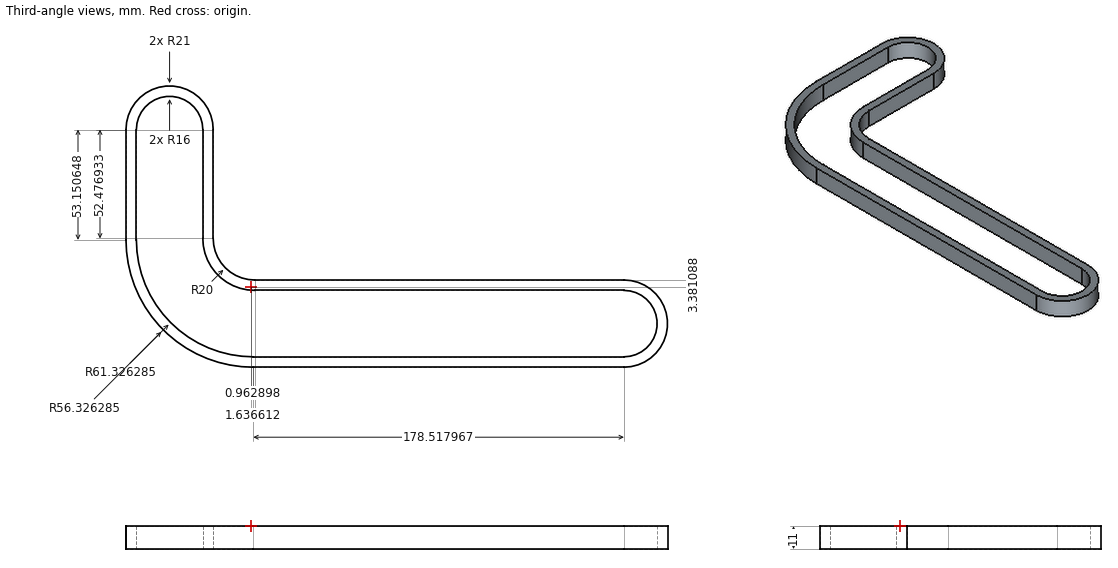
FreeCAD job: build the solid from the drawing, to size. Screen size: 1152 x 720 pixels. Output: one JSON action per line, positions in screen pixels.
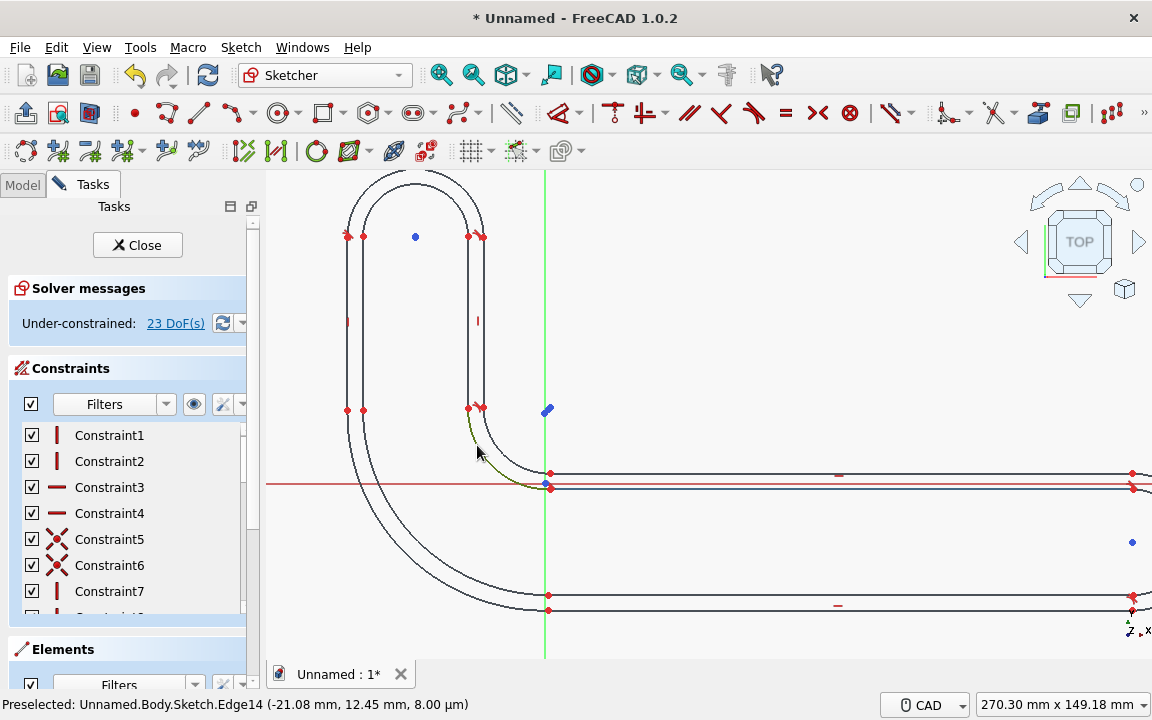
{"action": "left_click", "coordinate": [754, 114]}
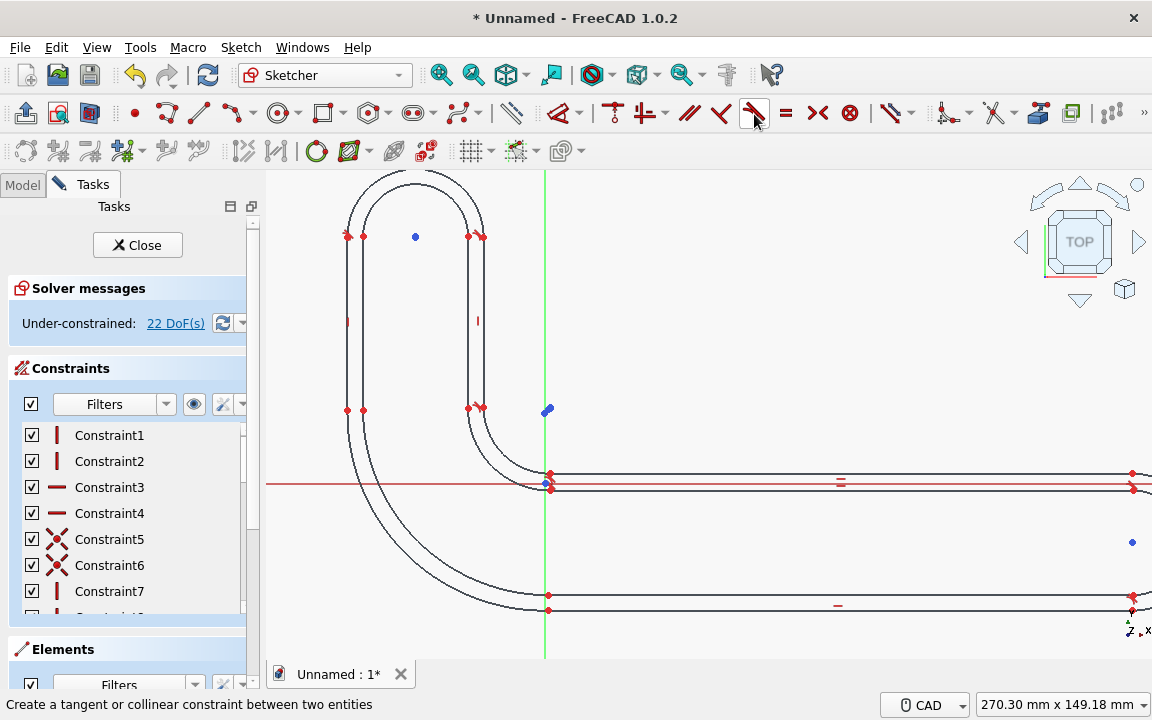
{"action": "scroll", "coordinate": [725, 491], "scroll_direction": "up", "scroll_amount": 4}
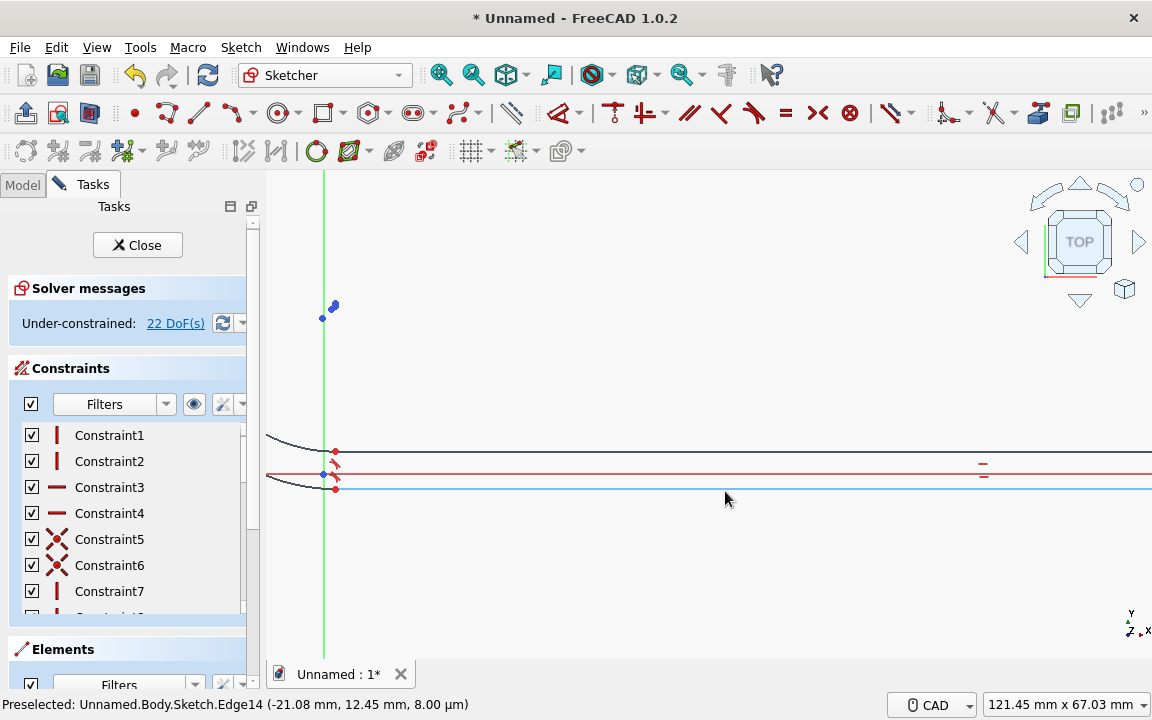
{"action": "left_click", "coordinate": [725, 489]}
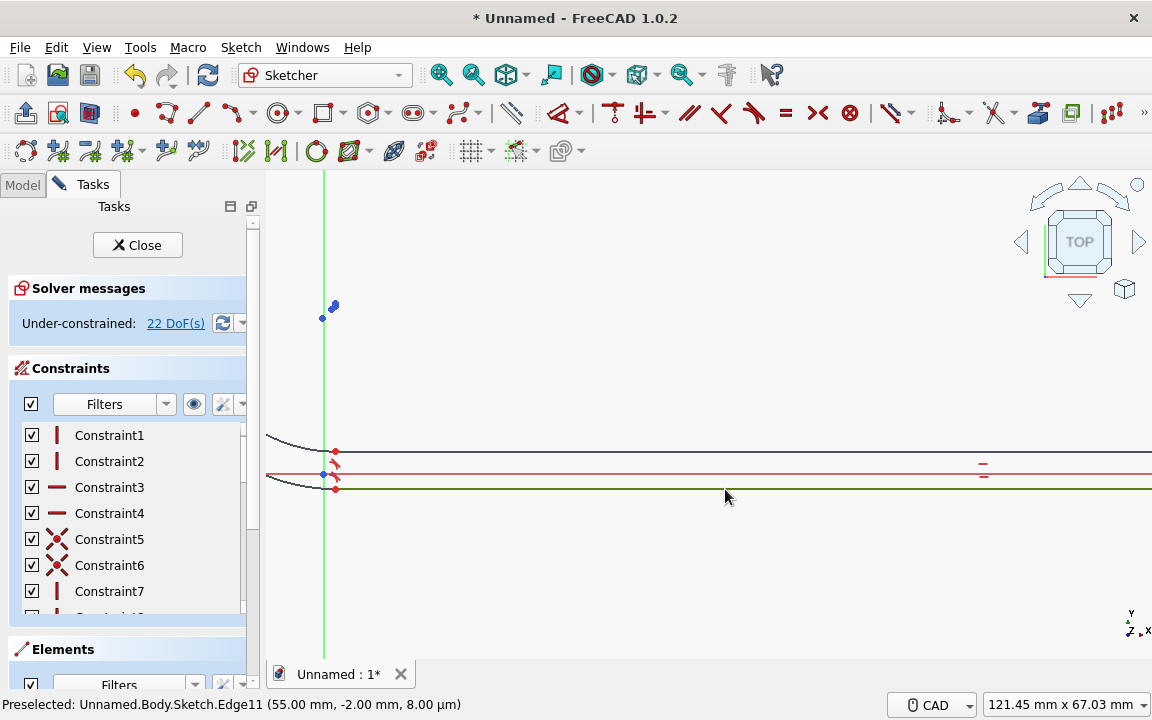
{"action": "scroll", "coordinate": [577, 464], "scroll_direction": "down", "scroll_amount": 7}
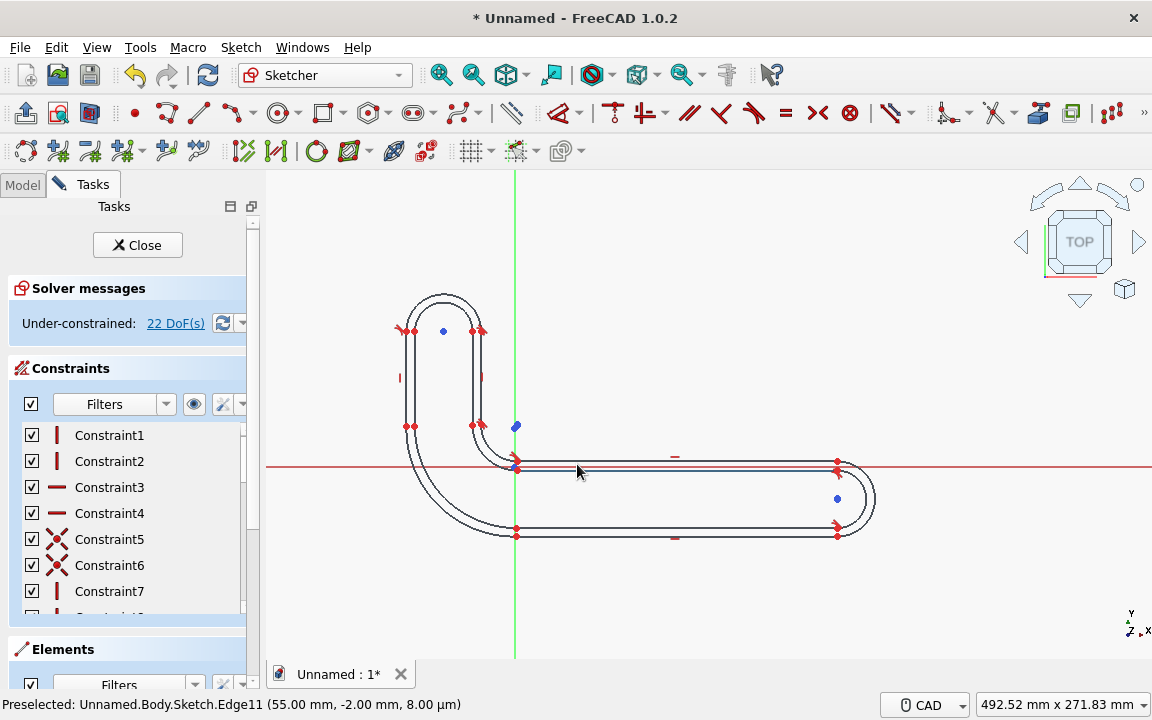
{"action": "scroll", "coordinate": [861, 516], "scroll_direction": "up", "scroll_amount": 3}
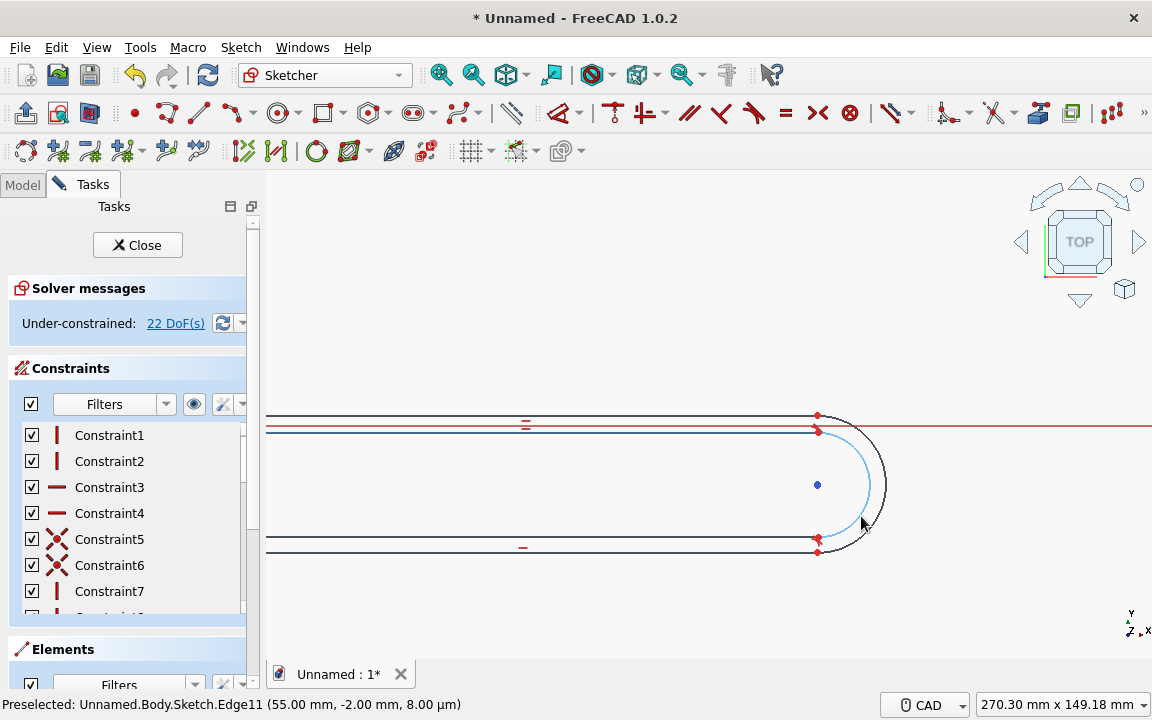
{"action": "left_click", "coordinate": [860, 516]}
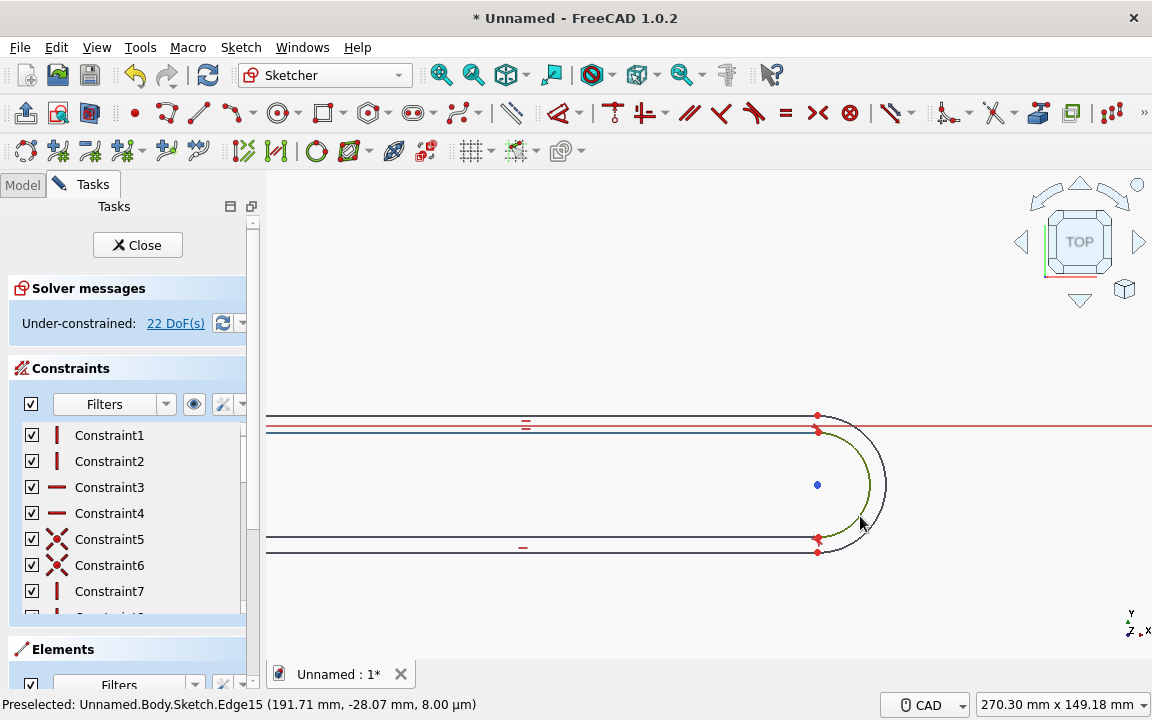
{"action": "left_click", "coordinate": [754, 114]}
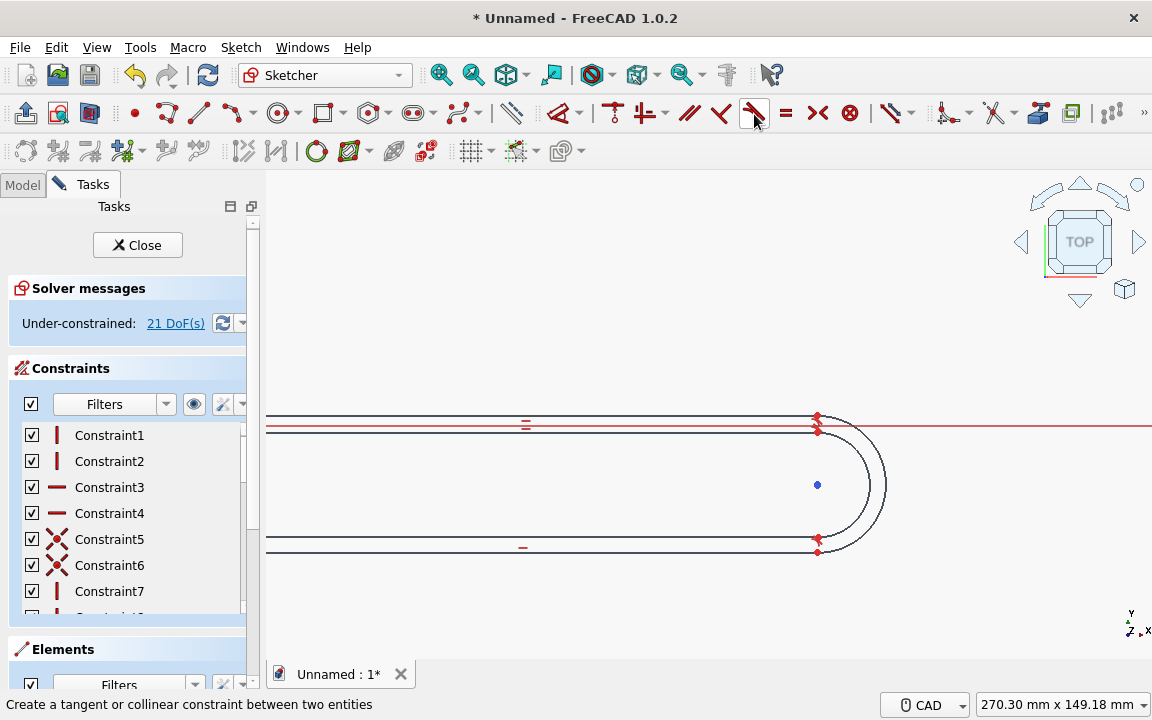
{"action": "left_click", "coordinate": [643, 537]}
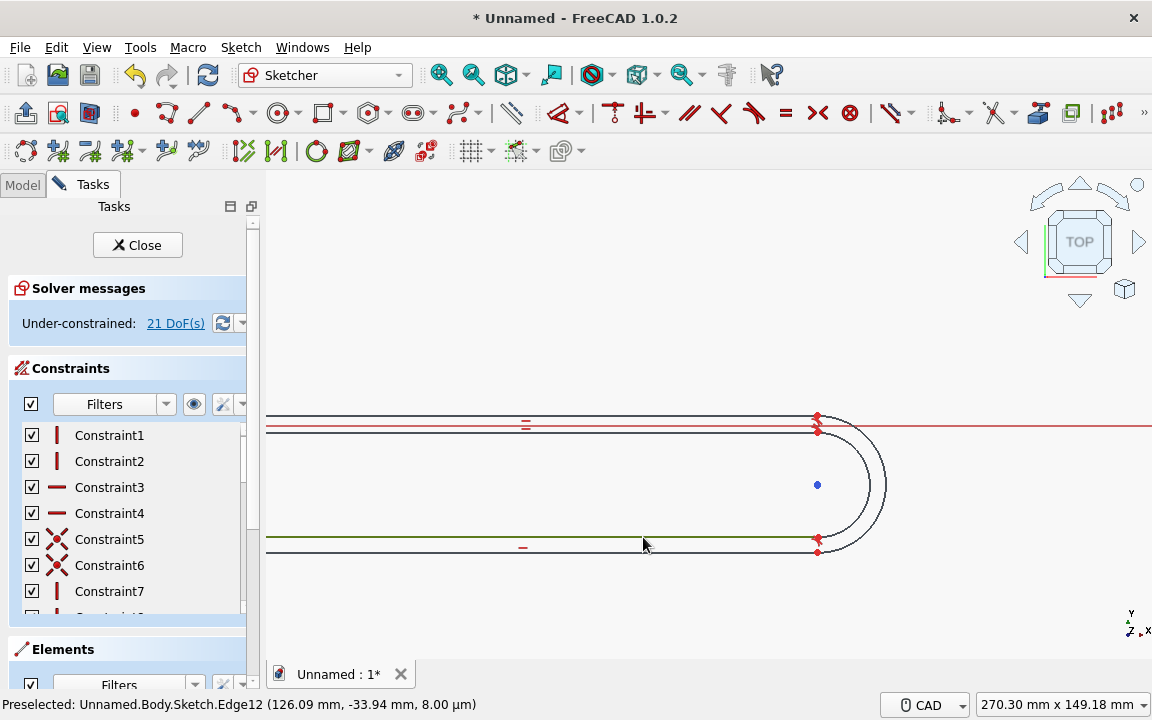
{"action": "left_click", "coordinate": [860, 516]}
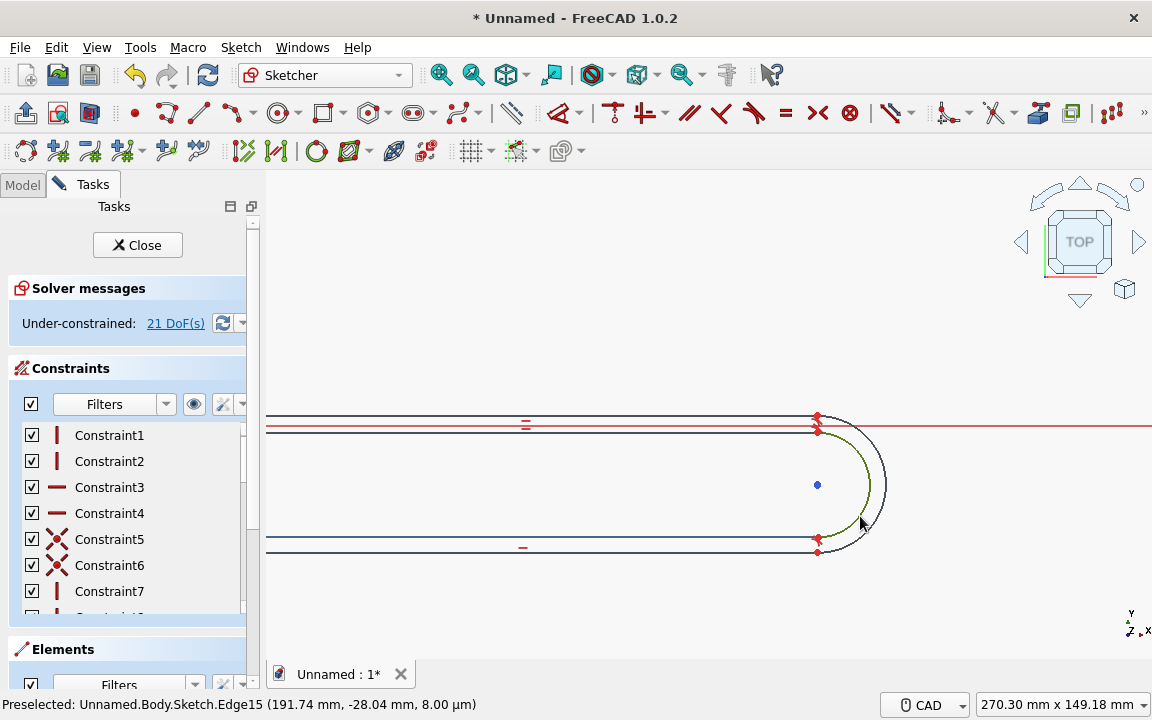
{"action": "left_click", "coordinate": [754, 114]}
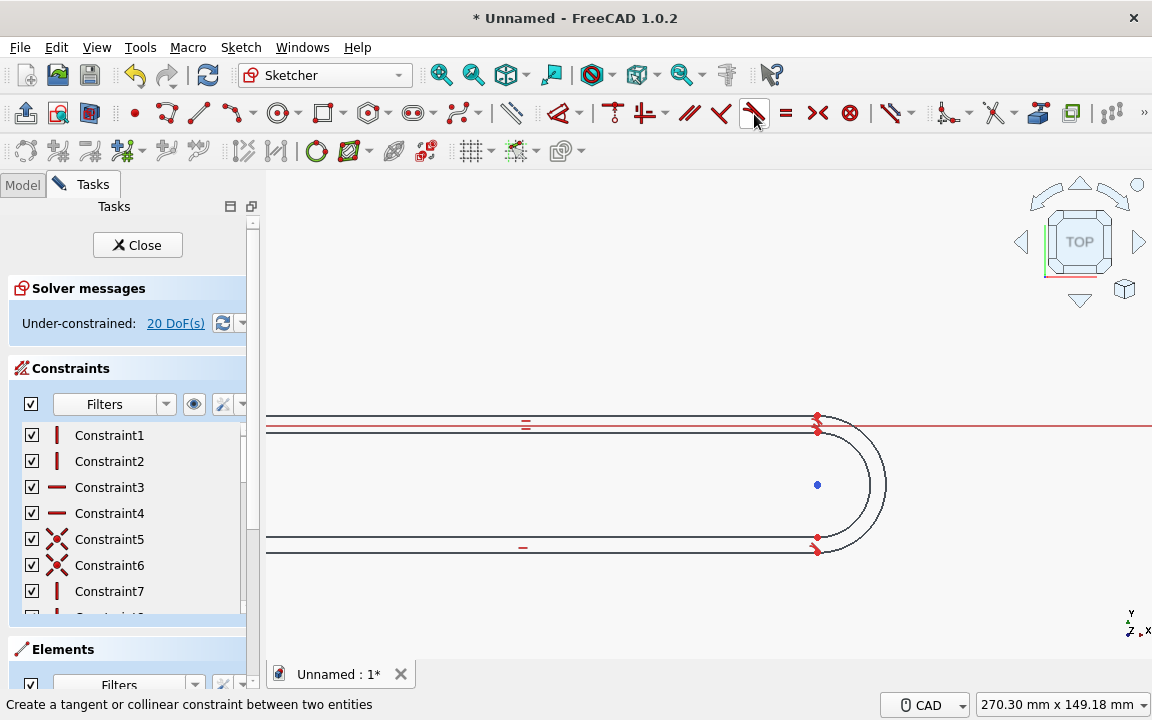
{"action": "scroll", "coordinate": [861, 516], "scroll_direction": "down", "scroll_amount": 3}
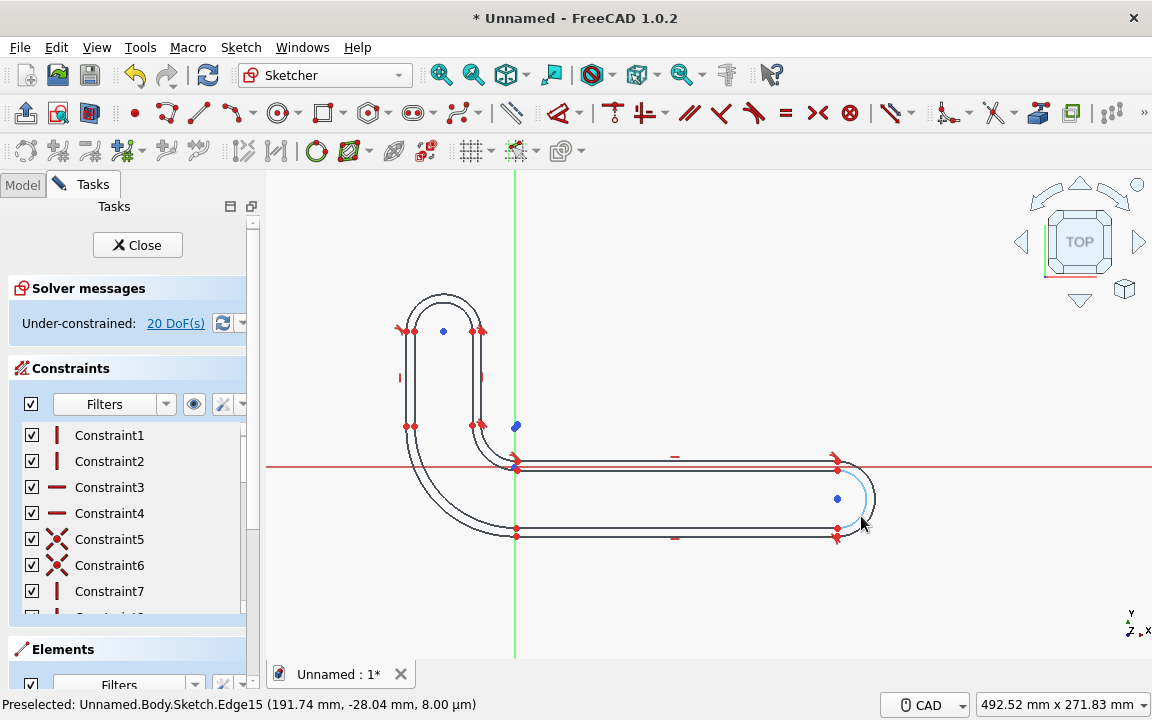
{"action": "scroll", "coordinate": [466, 301], "scroll_direction": "up", "scroll_amount": 3}